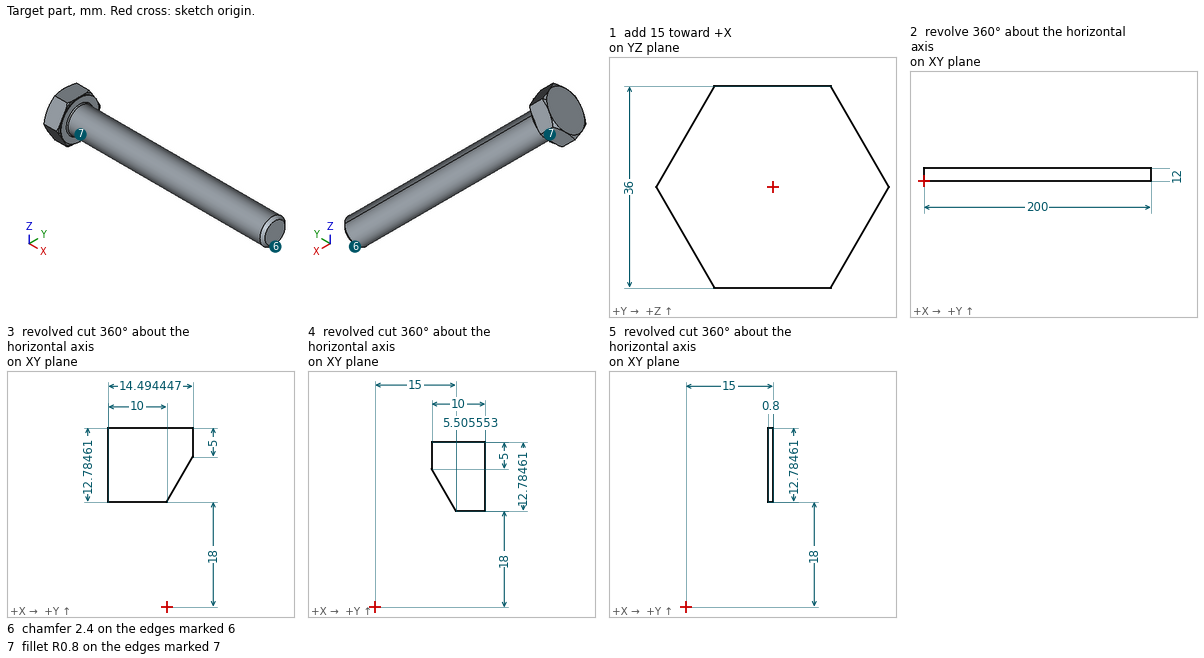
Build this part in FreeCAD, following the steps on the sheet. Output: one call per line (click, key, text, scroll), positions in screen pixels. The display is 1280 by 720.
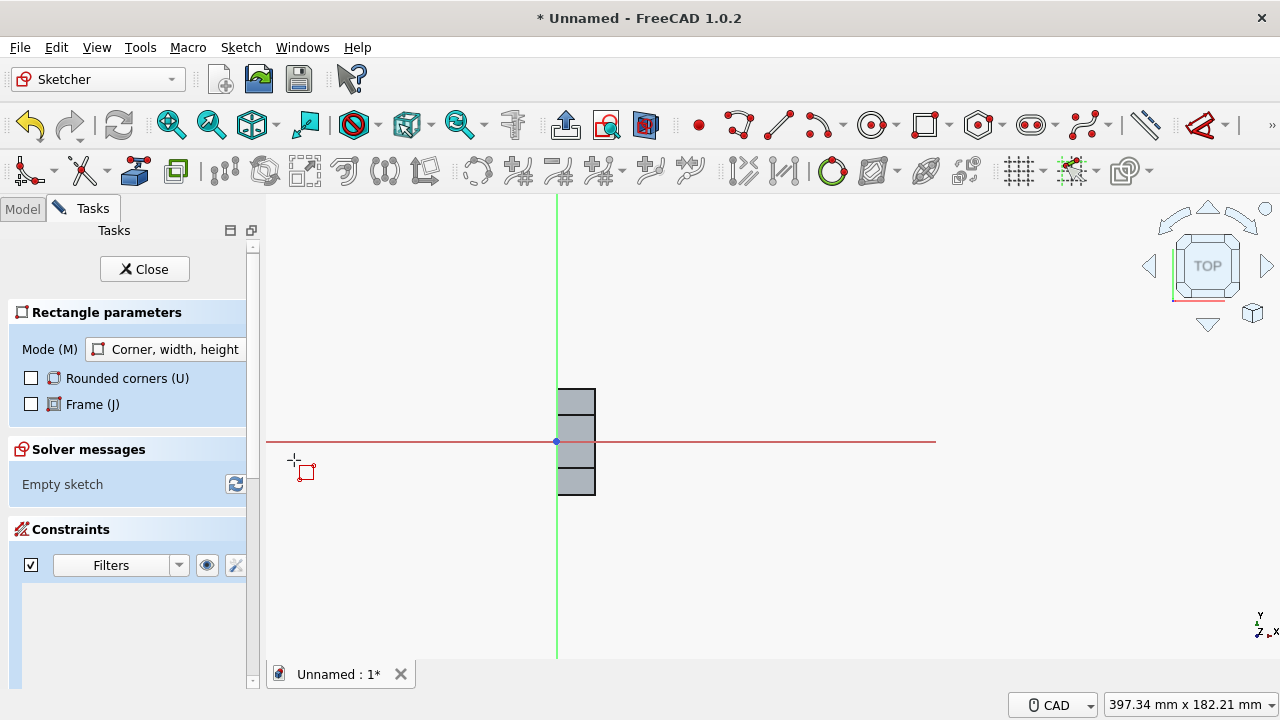
click(557, 442)
click(1067, 411)
key(Escape)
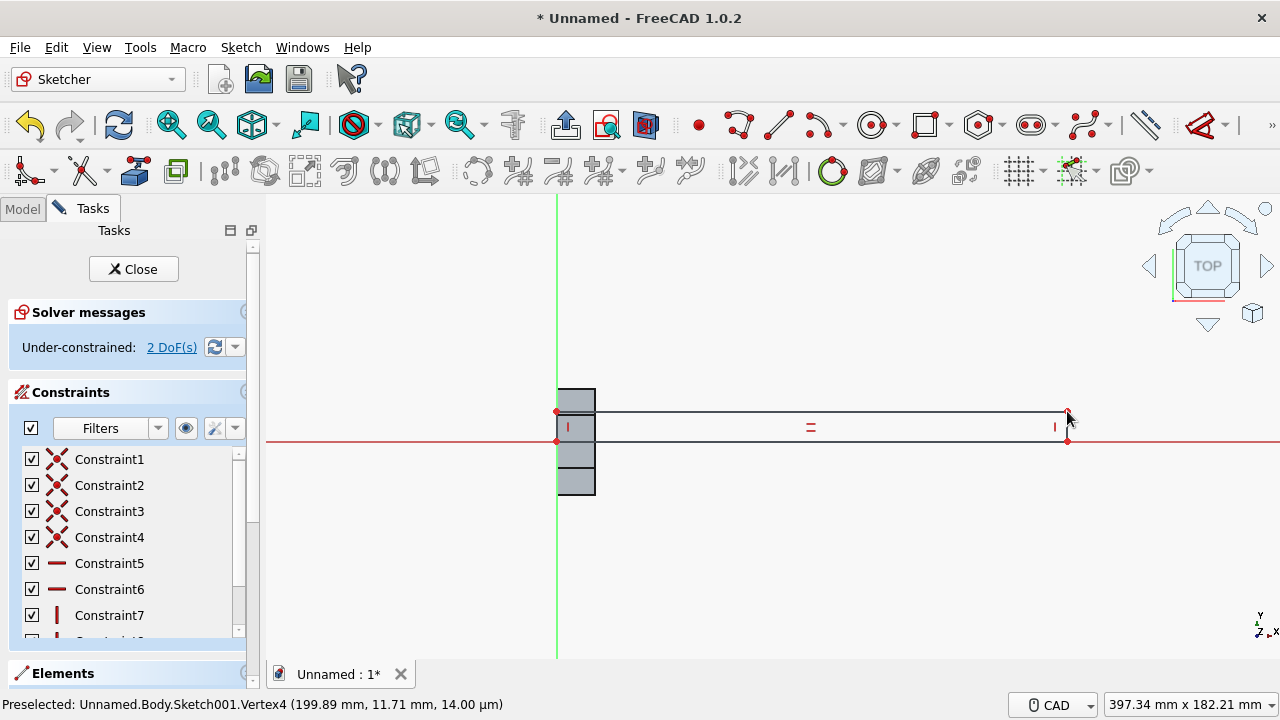
click(1200, 126)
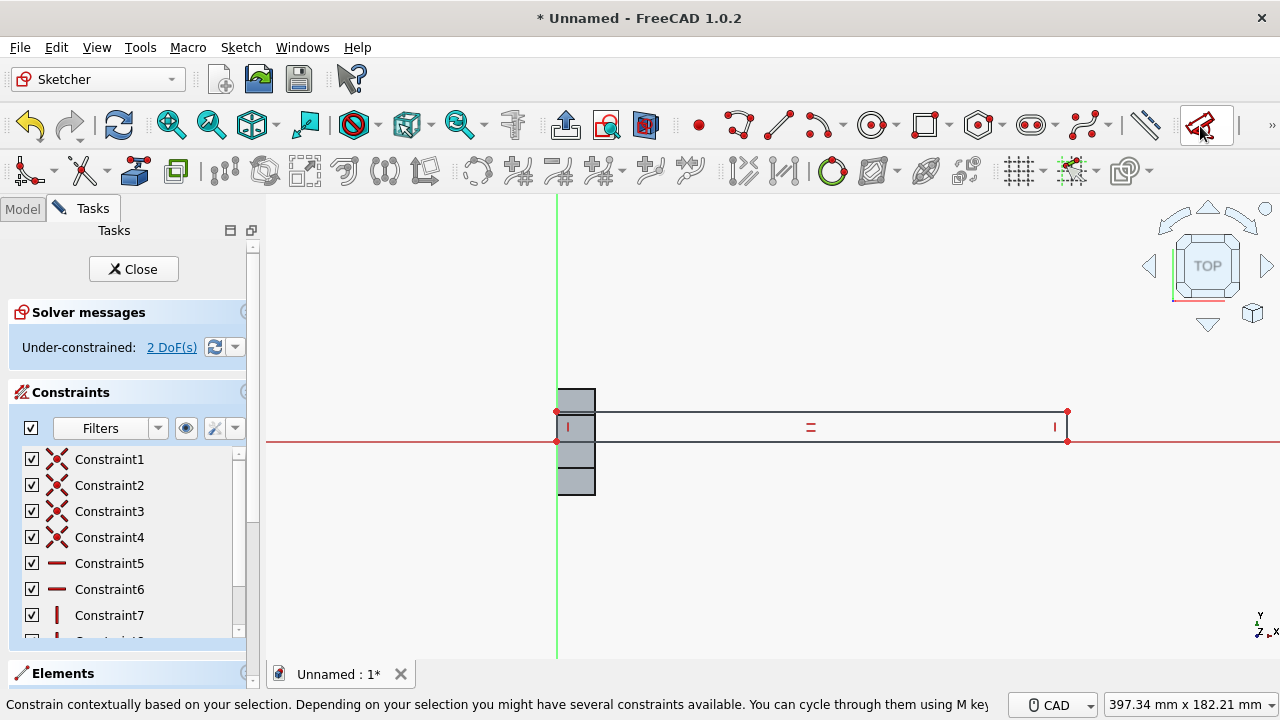
scroll(1067, 430, up, 2)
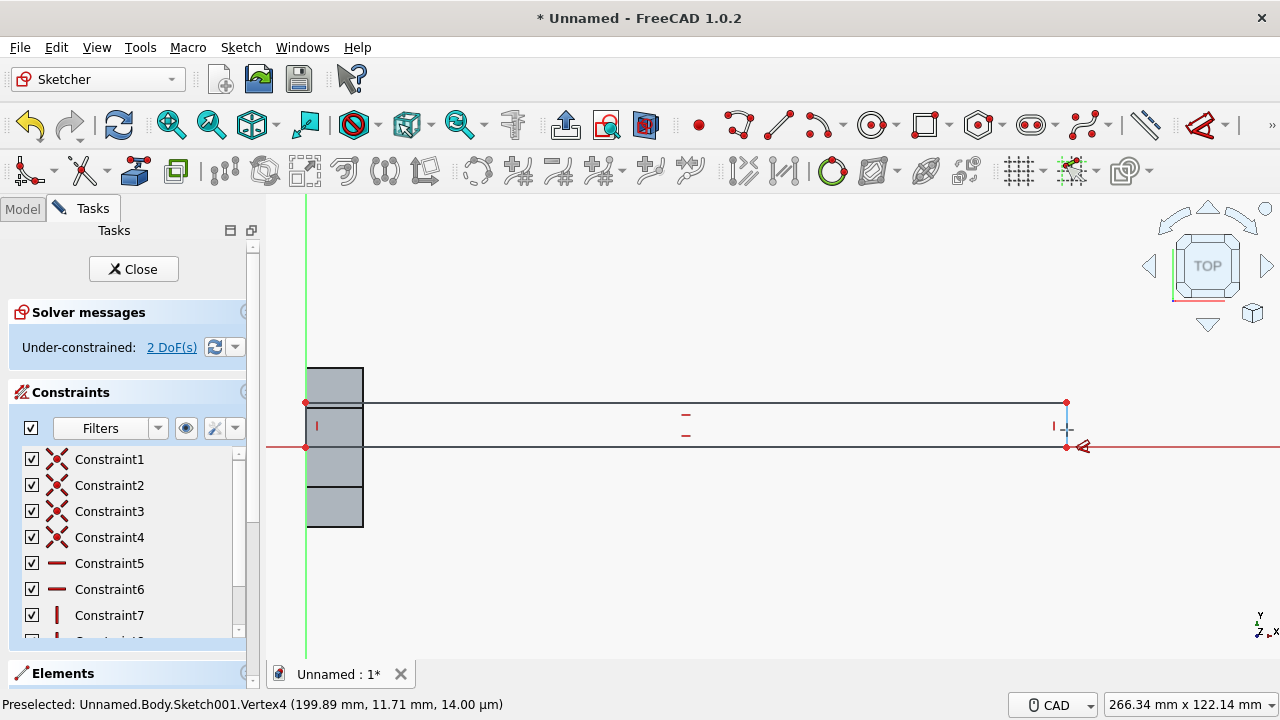
click(1067, 430)
click(1101, 425)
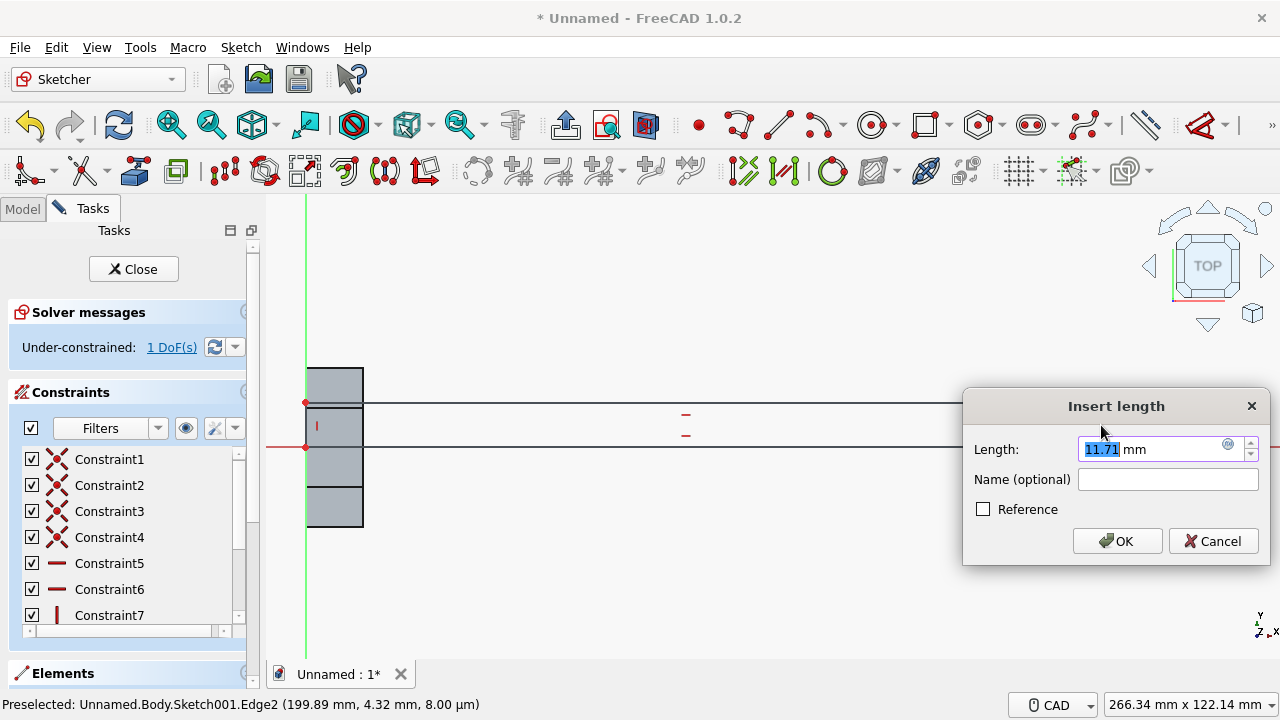
text(12)
key(Return)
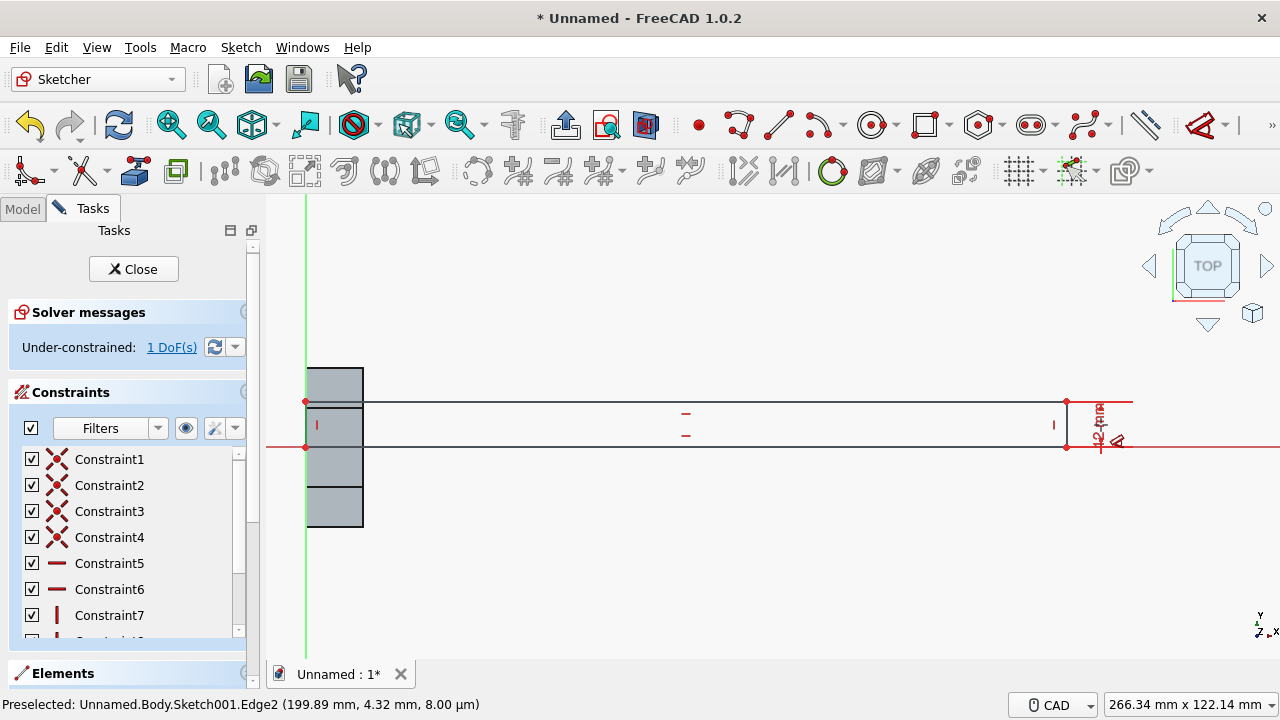
click(534, 447)
click(686, 481)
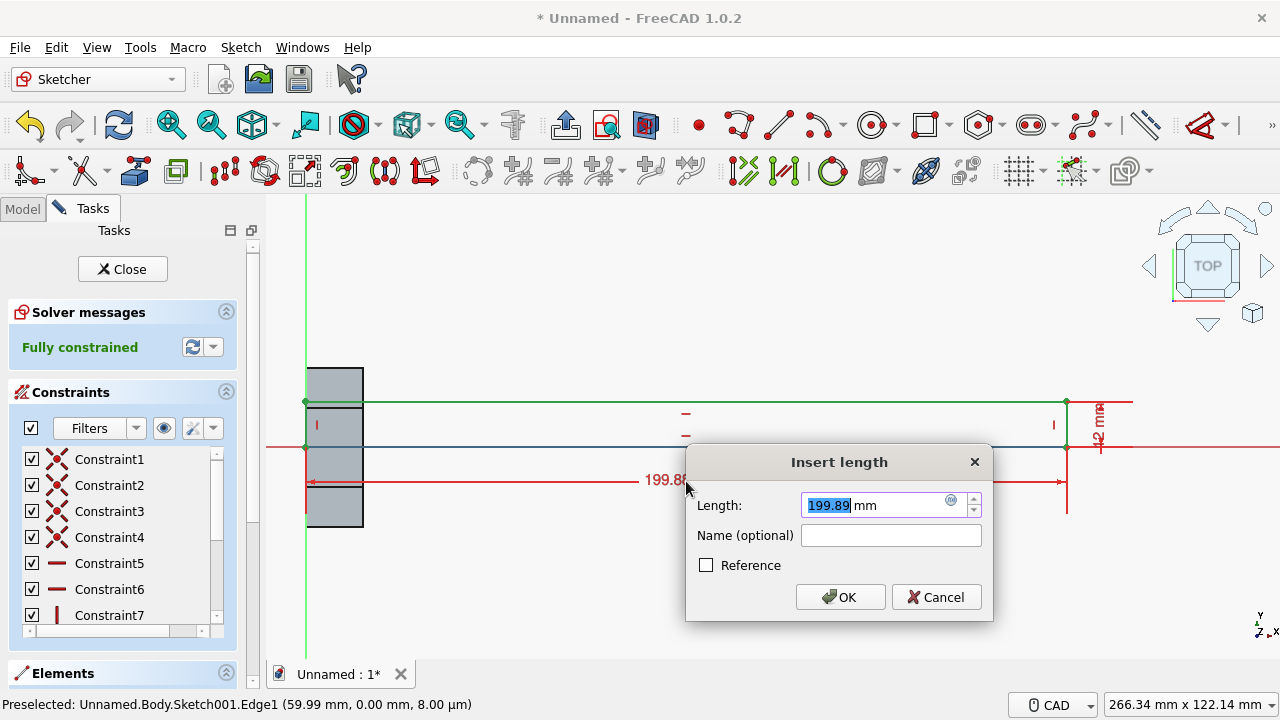
text(200)
key(Return)
key(Escape)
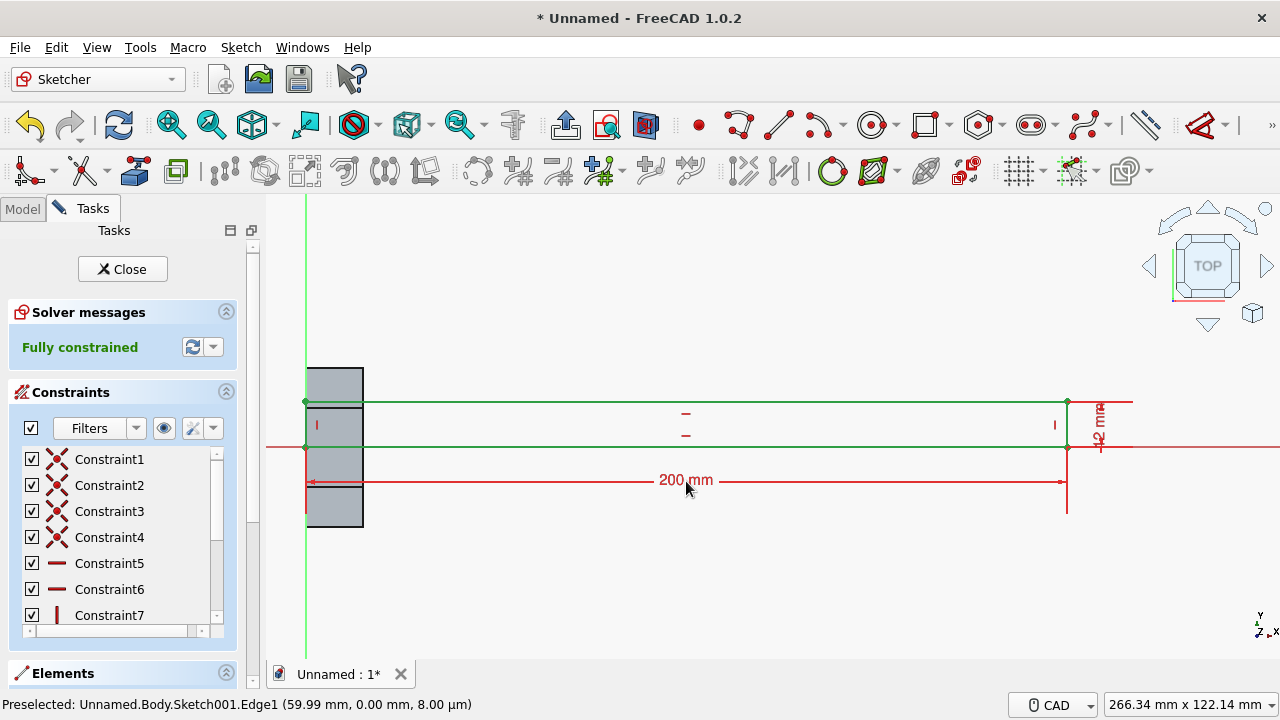
click(123, 269)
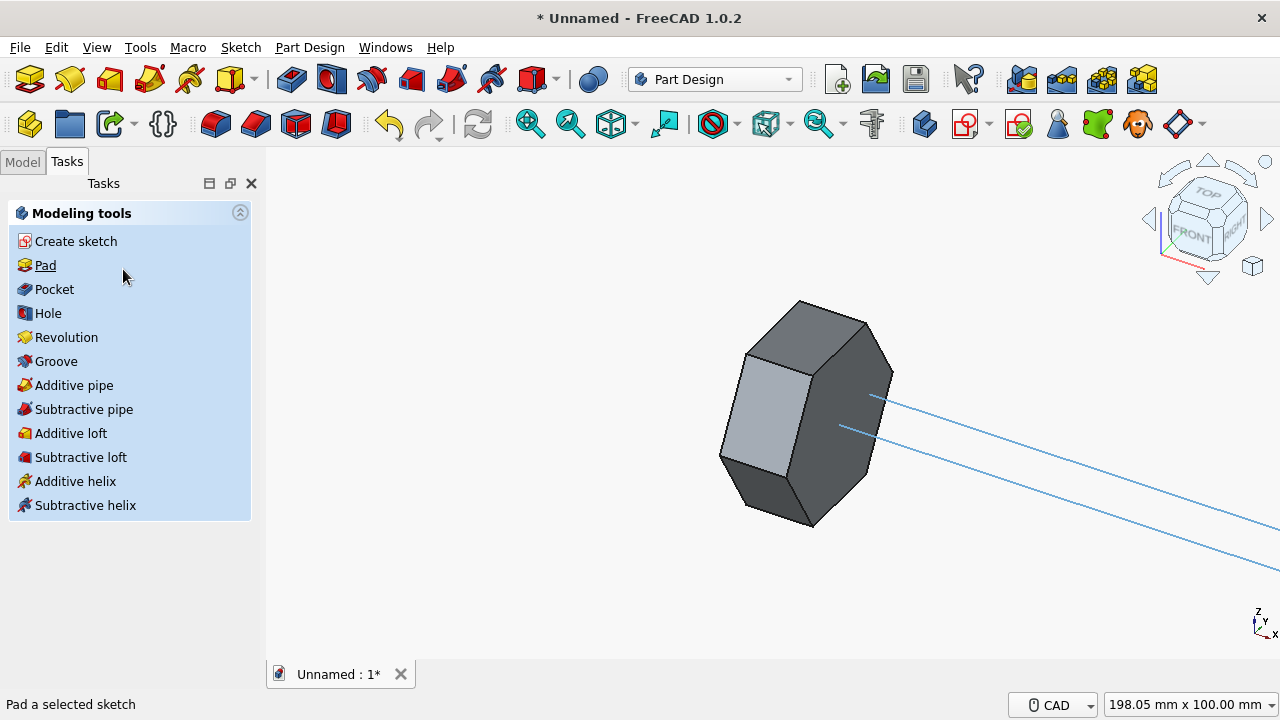
click(70, 80)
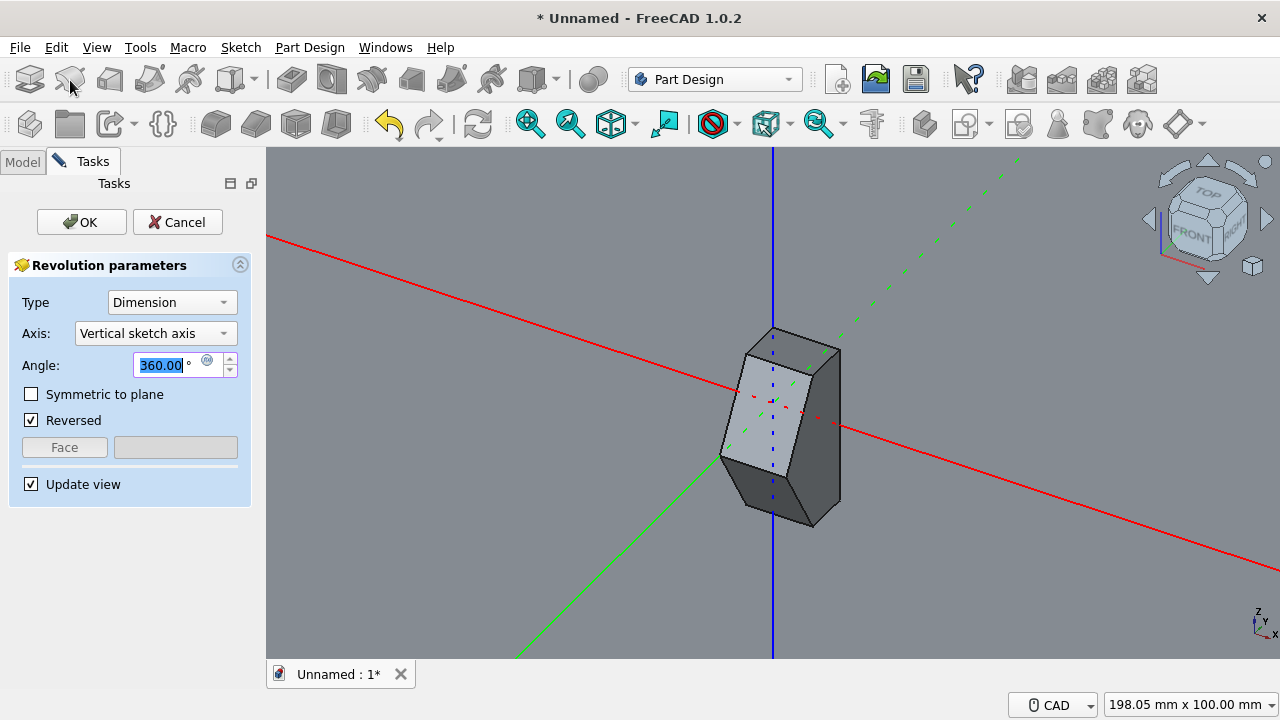
click(156, 334)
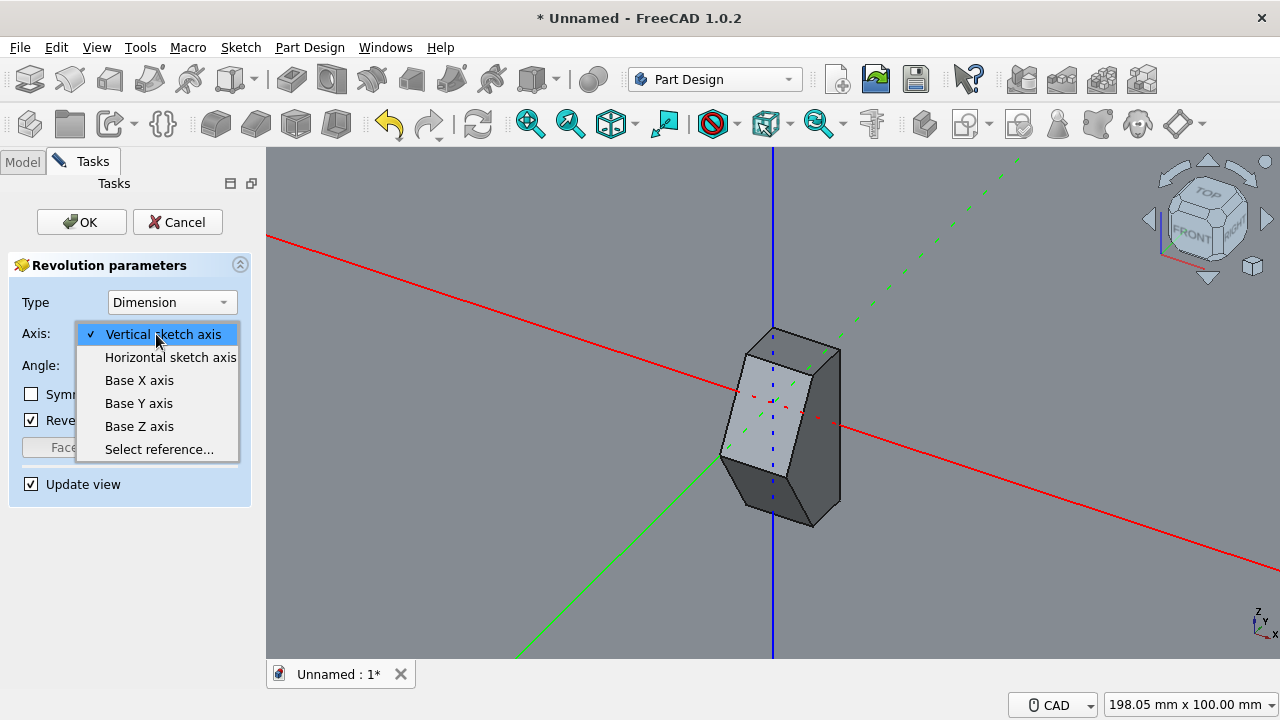
click(156, 358)